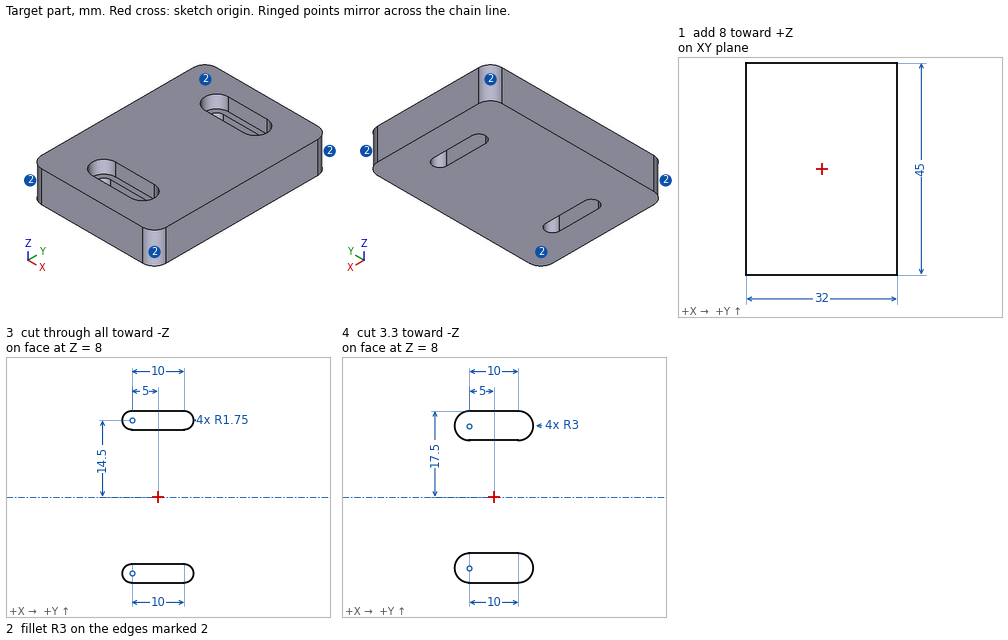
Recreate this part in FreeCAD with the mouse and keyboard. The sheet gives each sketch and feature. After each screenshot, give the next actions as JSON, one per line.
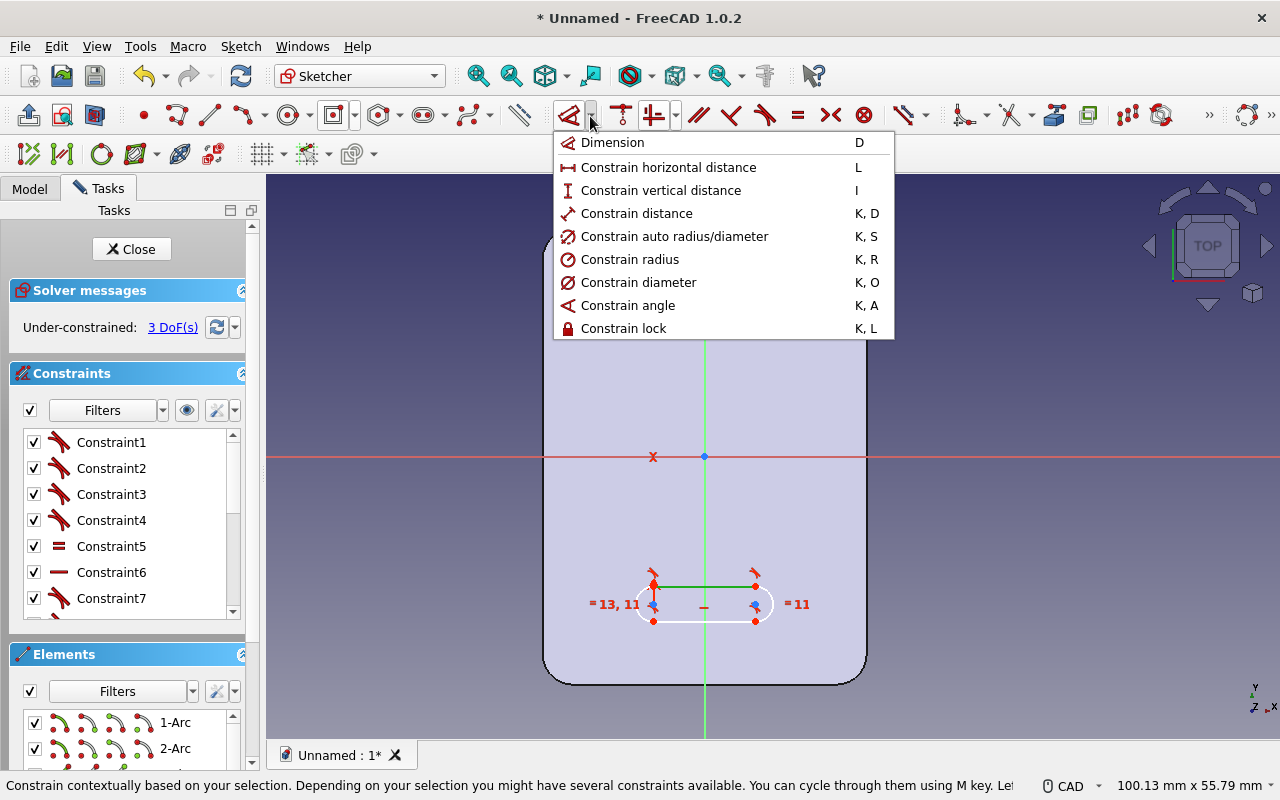
{"action": "left_click", "coordinate": [724, 168]}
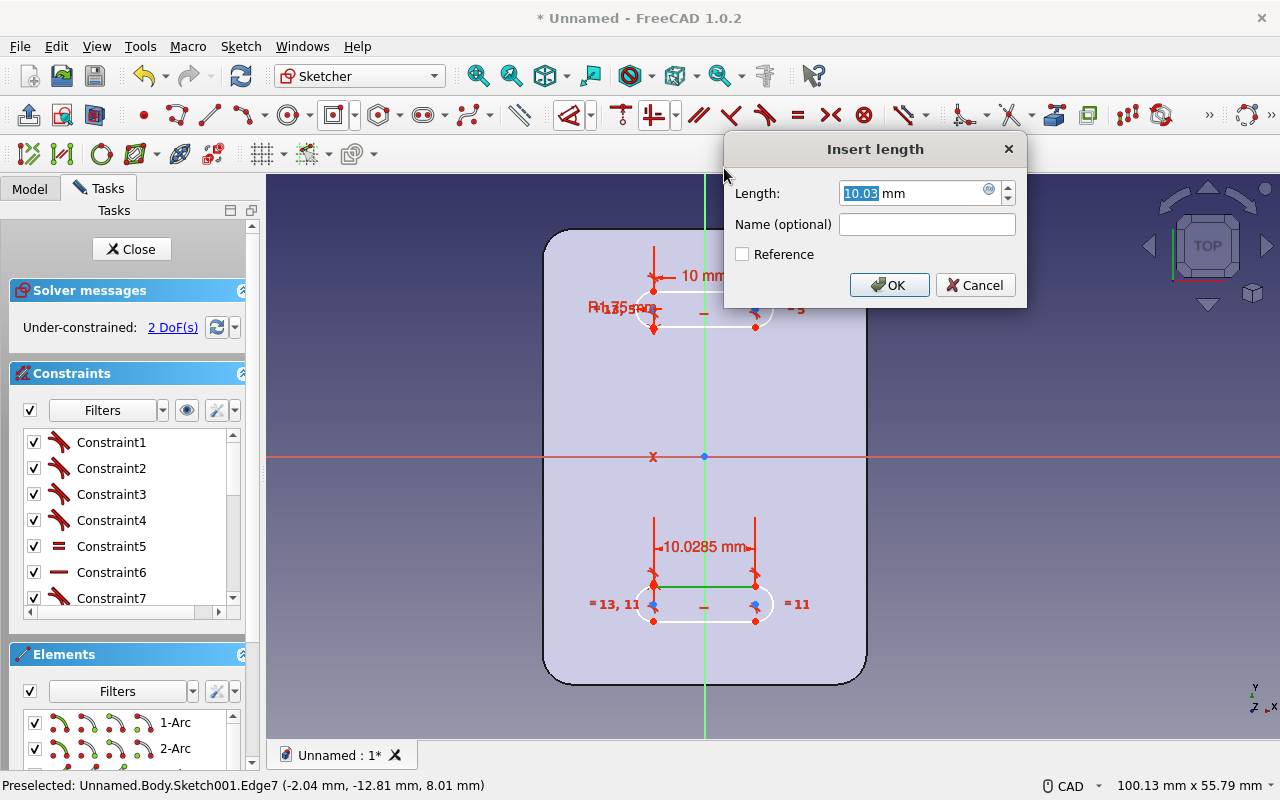
{"action": "type", "text": "10"}
{"action": "key", "text": "Return"}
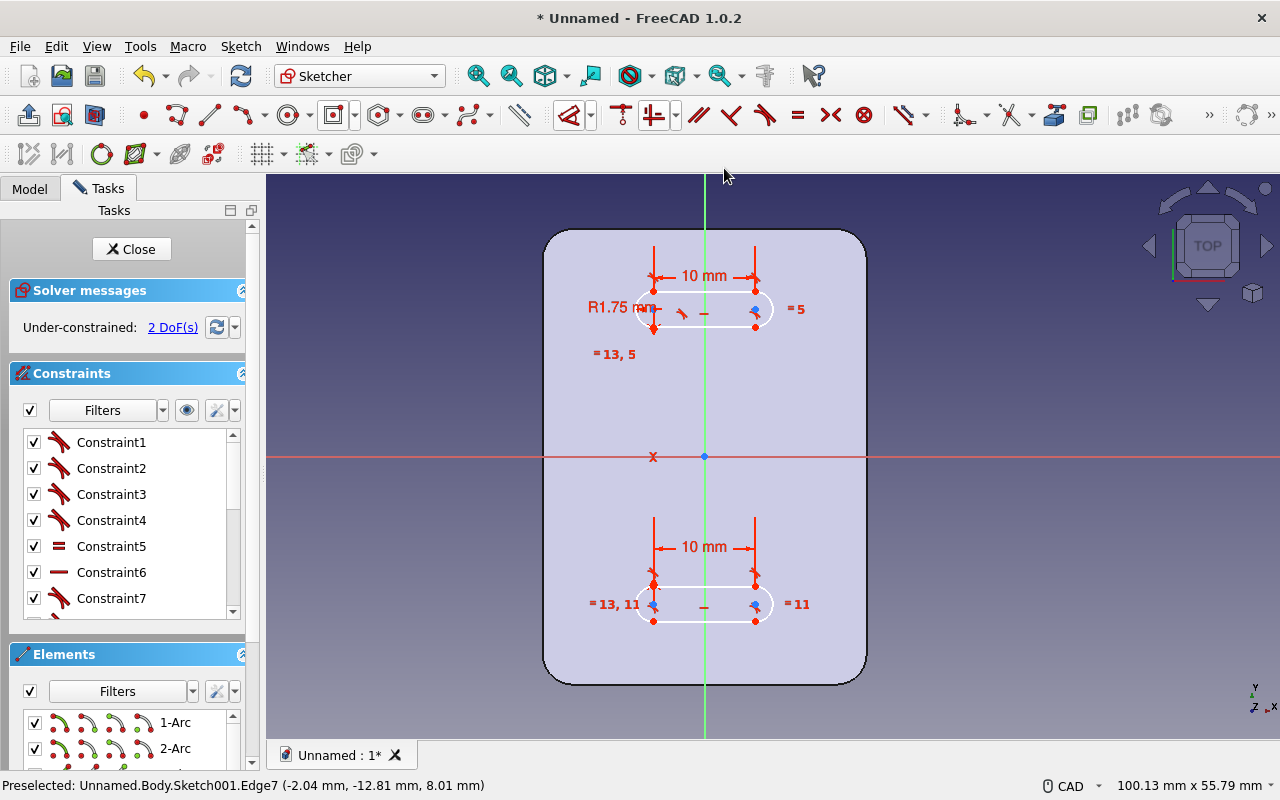
{"action": "left_click", "coordinate": [654, 292]}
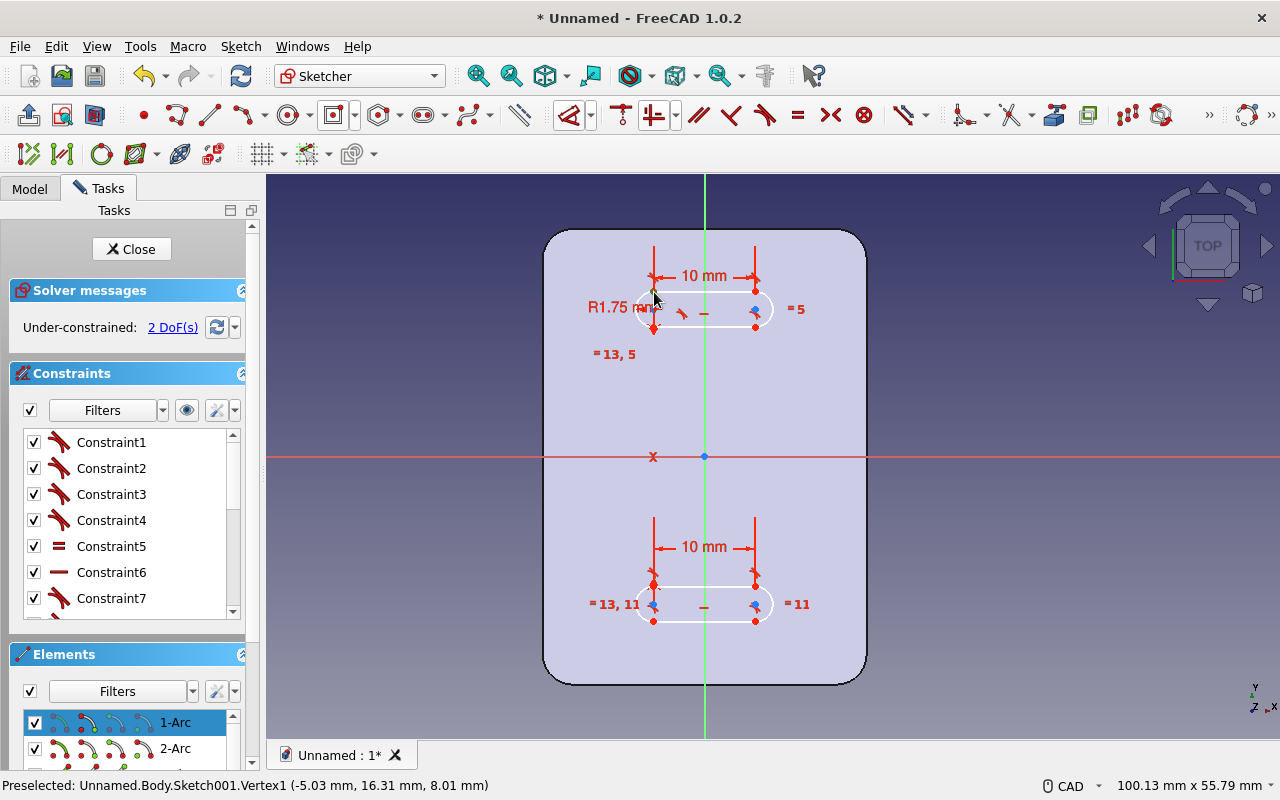
{"action": "key", "text": "l"}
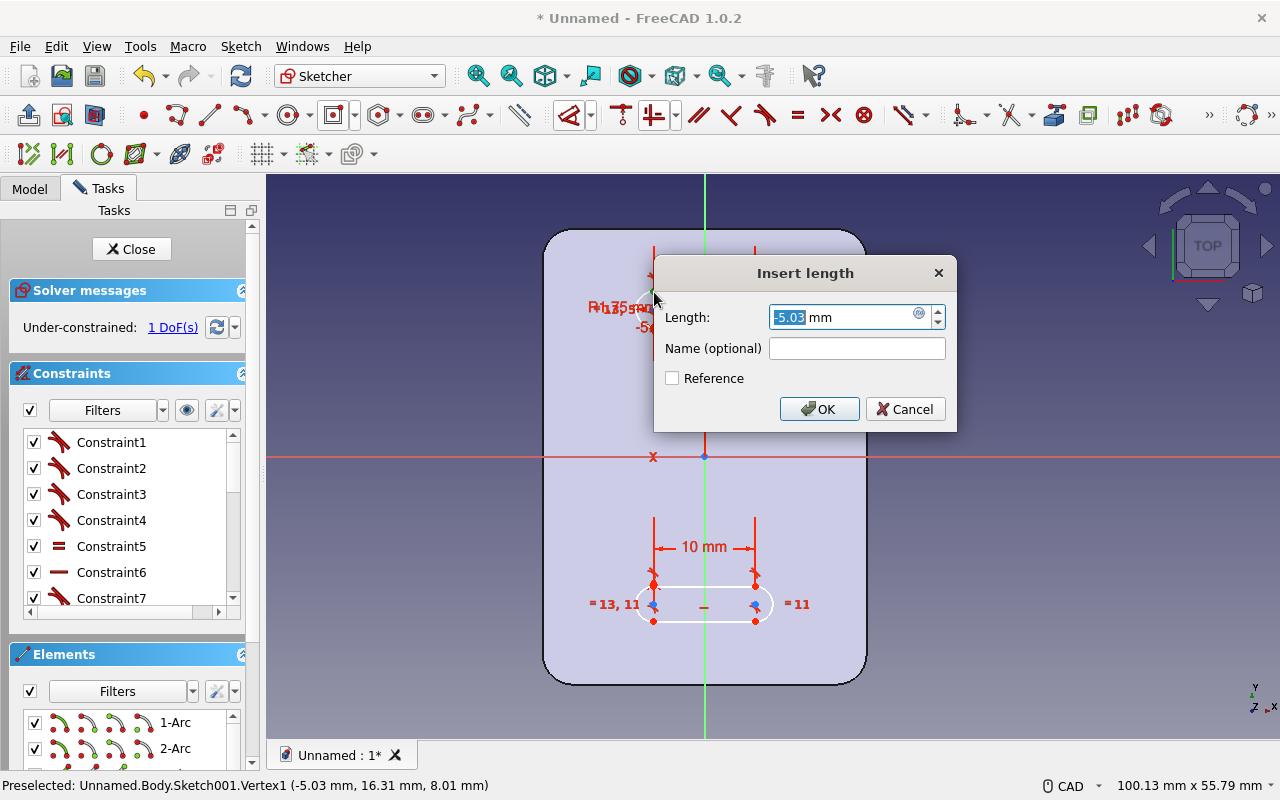
{"action": "type", "text": "-5"}
{"action": "key", "text": "Return"}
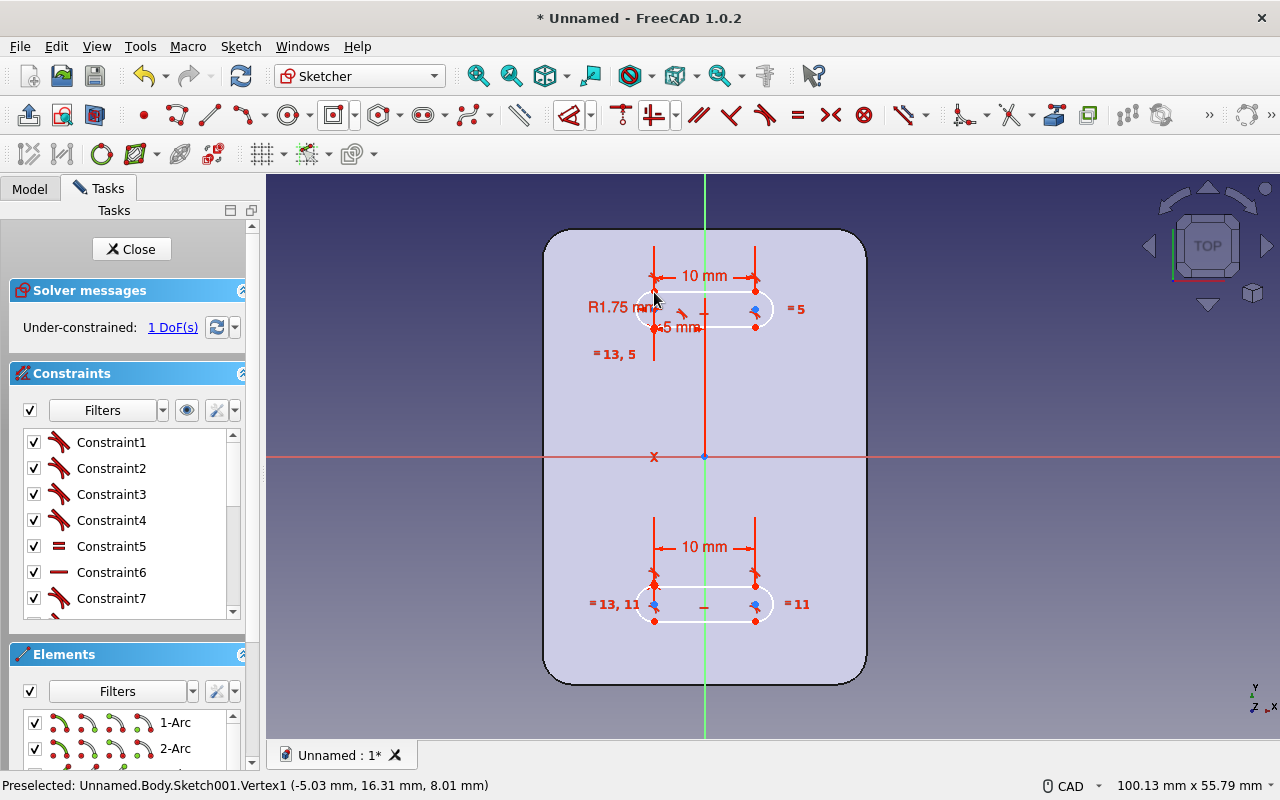
{"action": "left_click", "coordinate": [654, 309]}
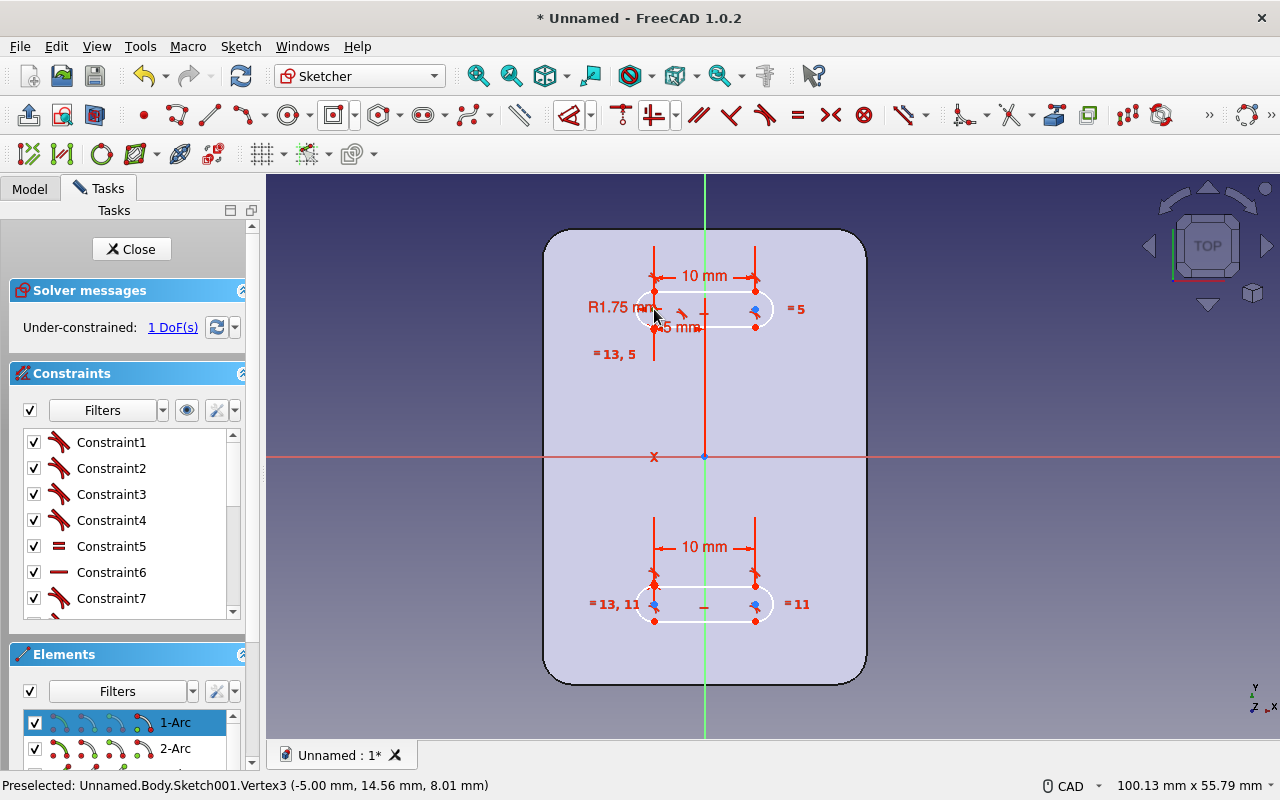
{"action": "key", "text": "i"}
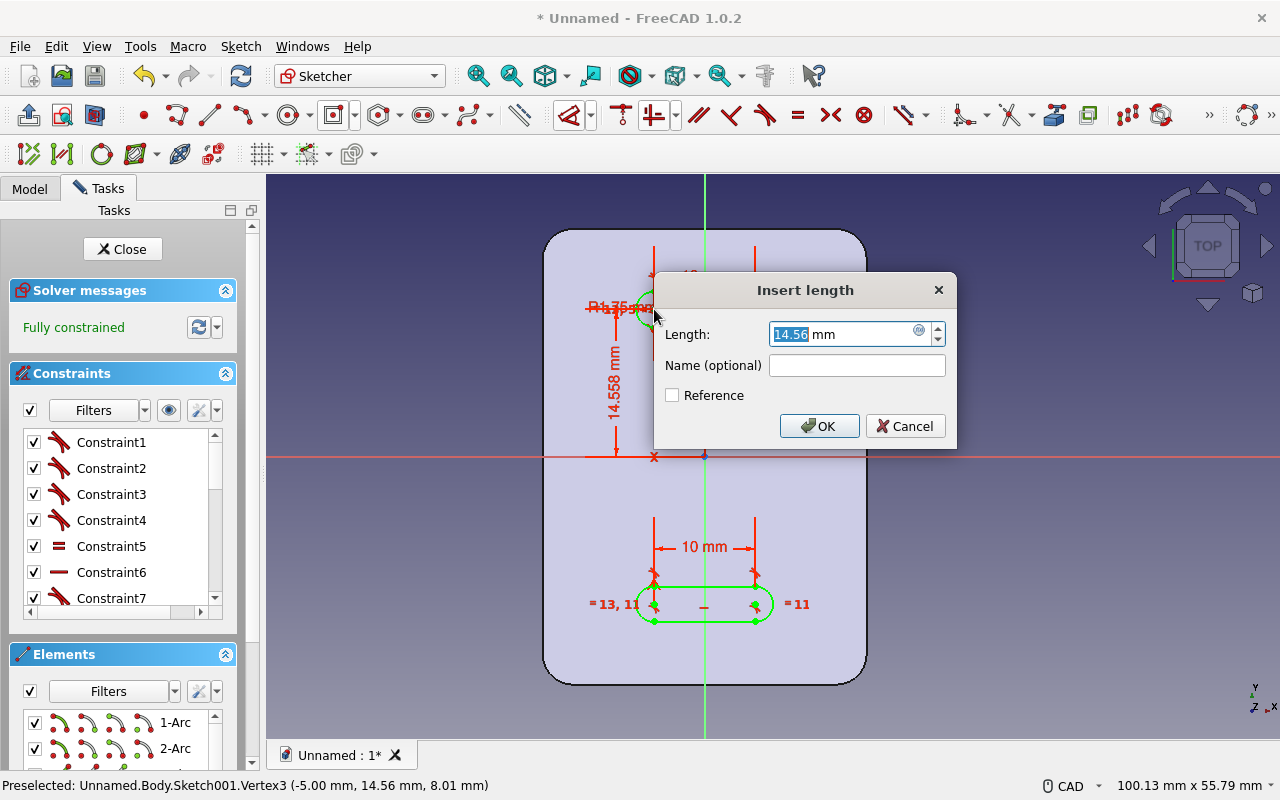
{"action": "type", "text": "14.5"}
{"action": "key", "text": "Return"}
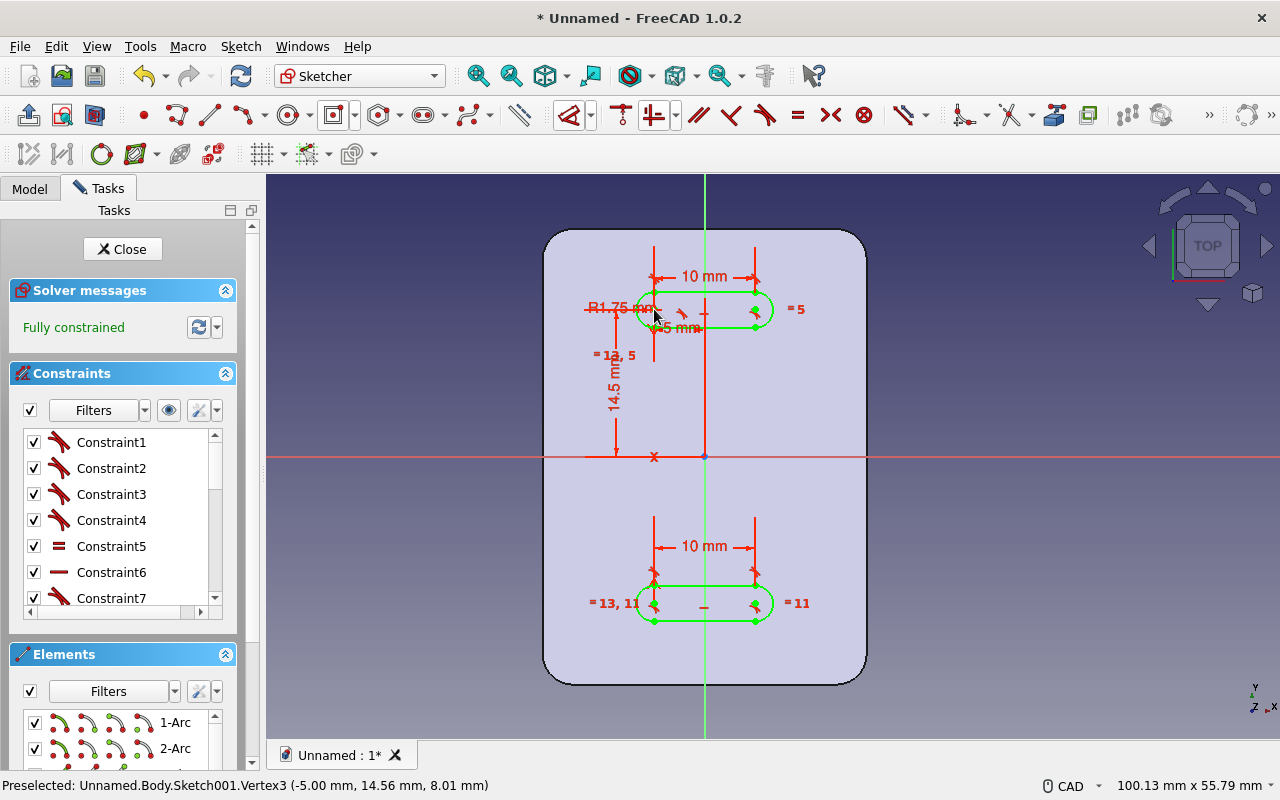
{"action": "left_click", "coordinate": [123, 249]}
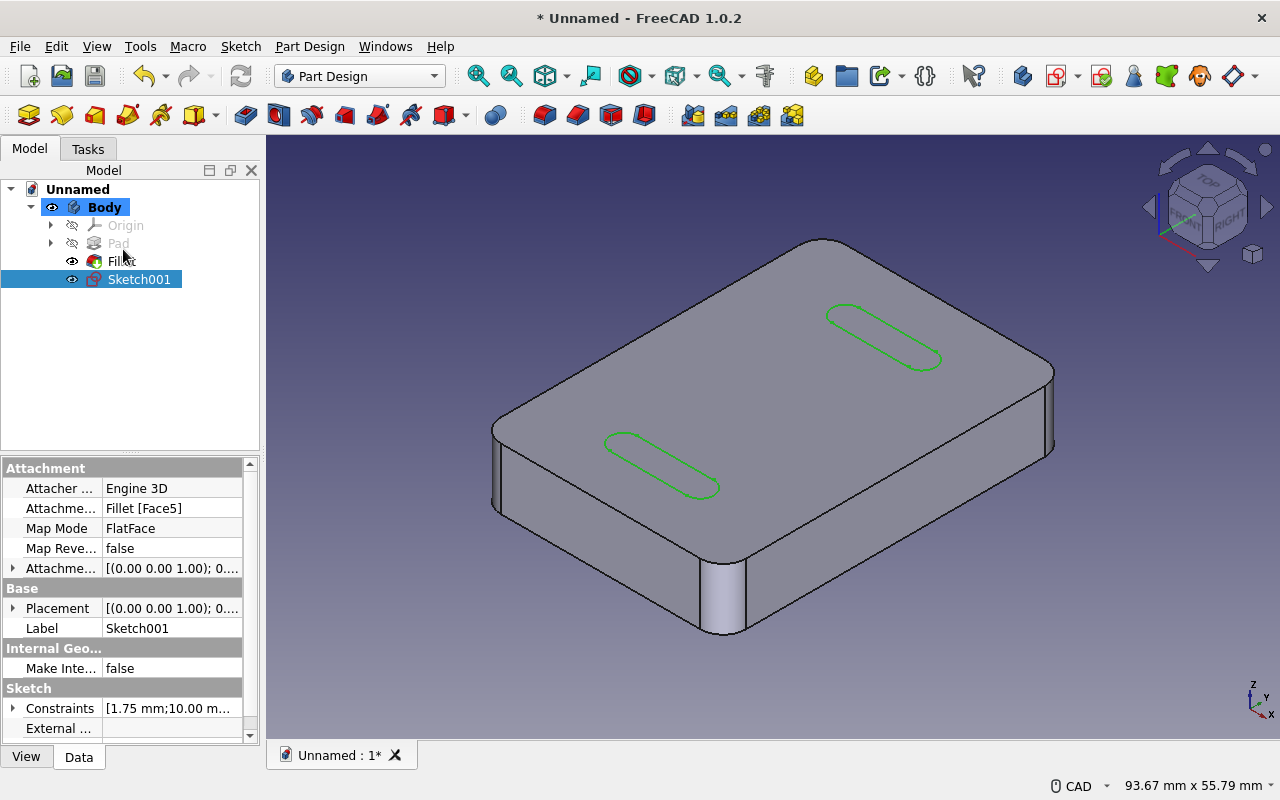
{"action": "left_click", "coordinate": [246, 116]}